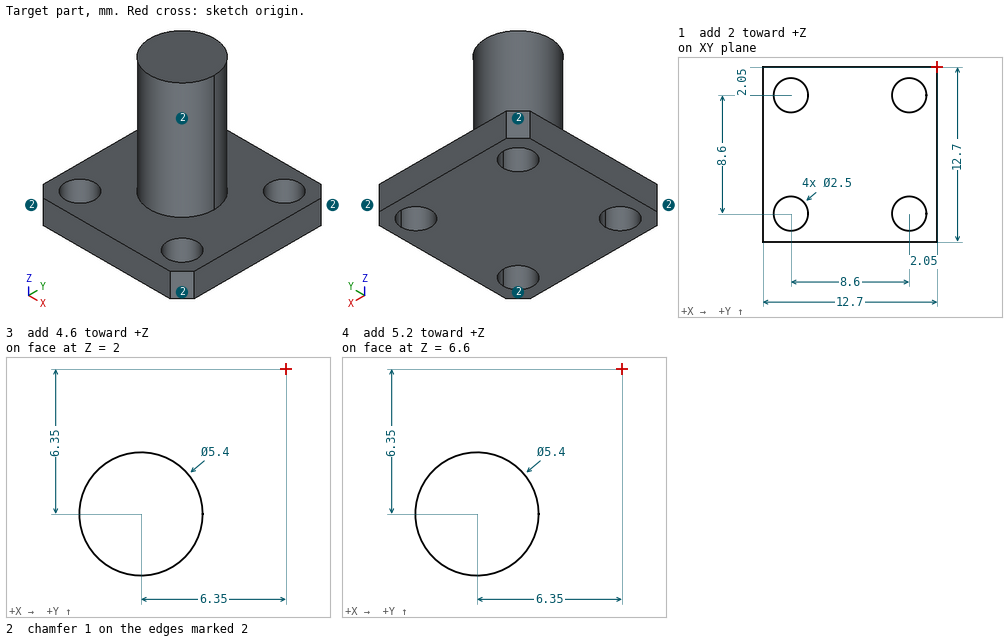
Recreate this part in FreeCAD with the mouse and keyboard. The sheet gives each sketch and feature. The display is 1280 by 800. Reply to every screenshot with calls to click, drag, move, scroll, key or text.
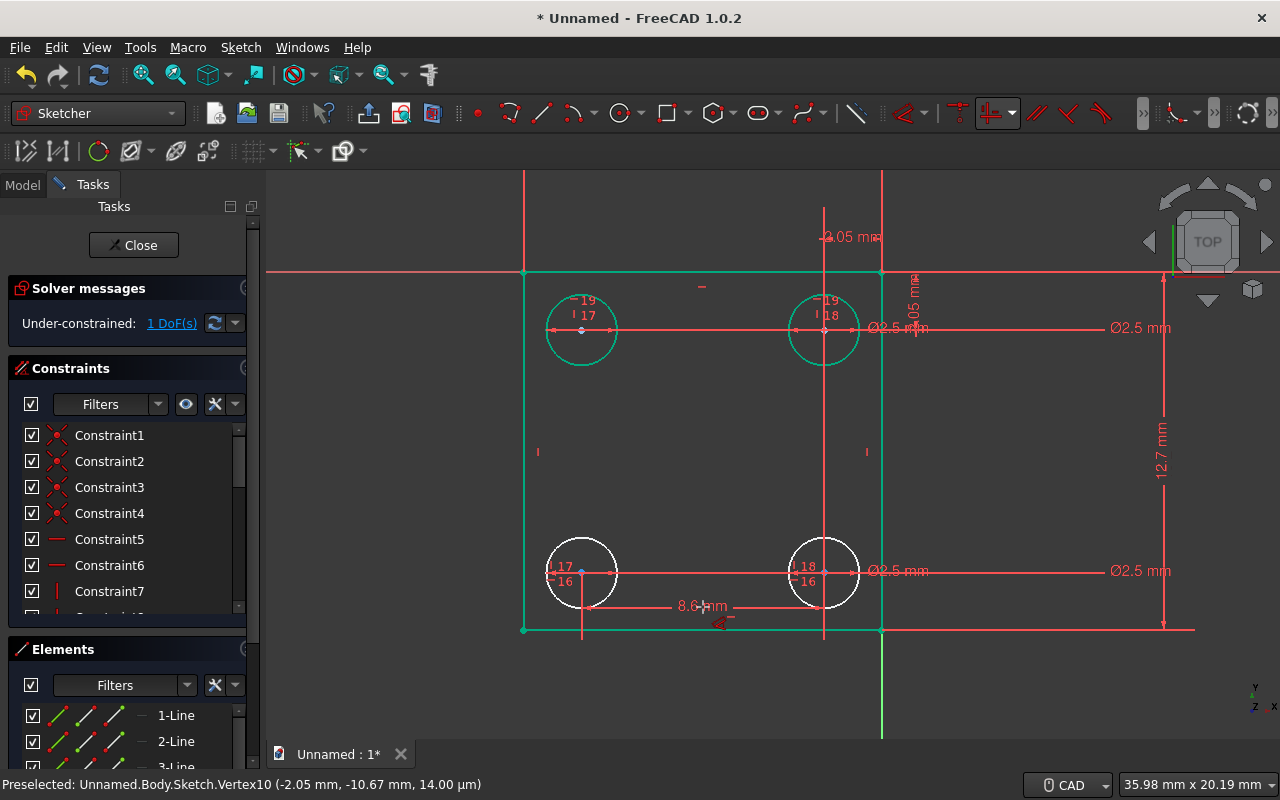
click(582, 573)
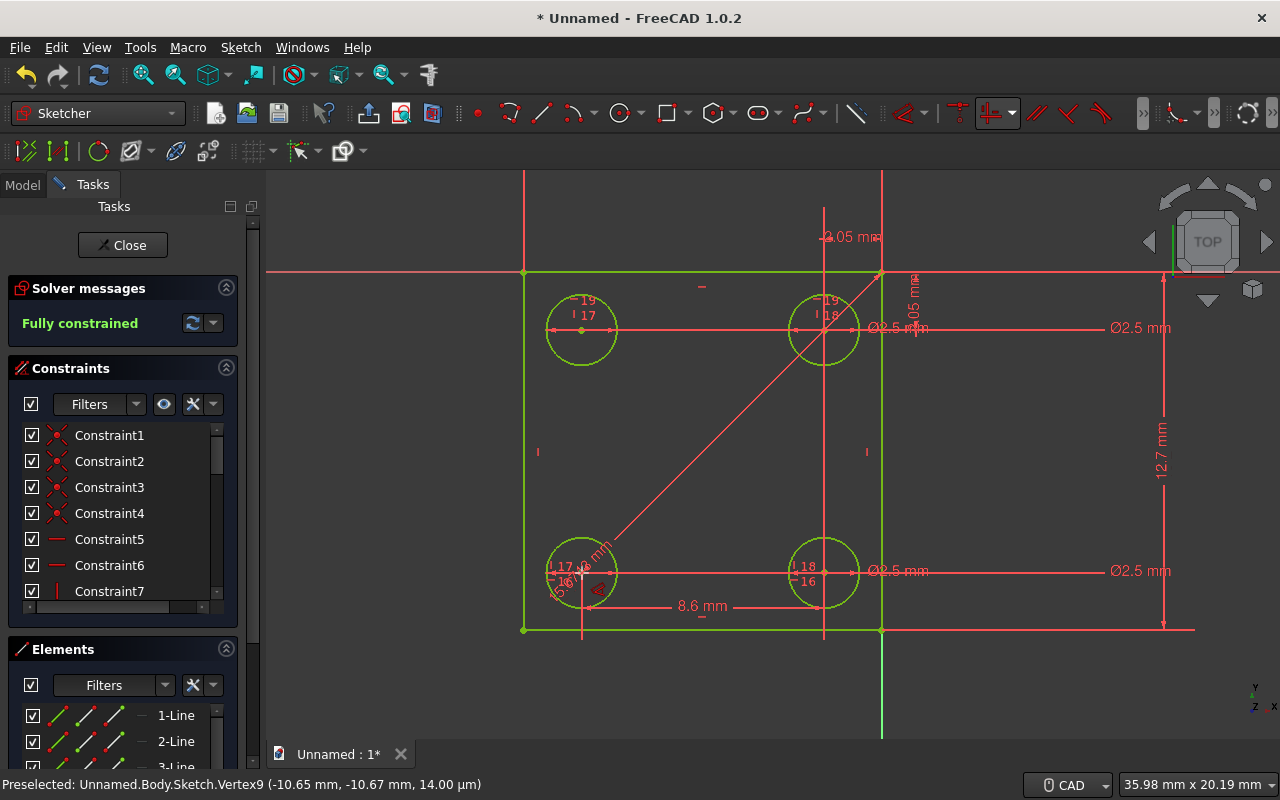
click(582, 330)
click(548, 452)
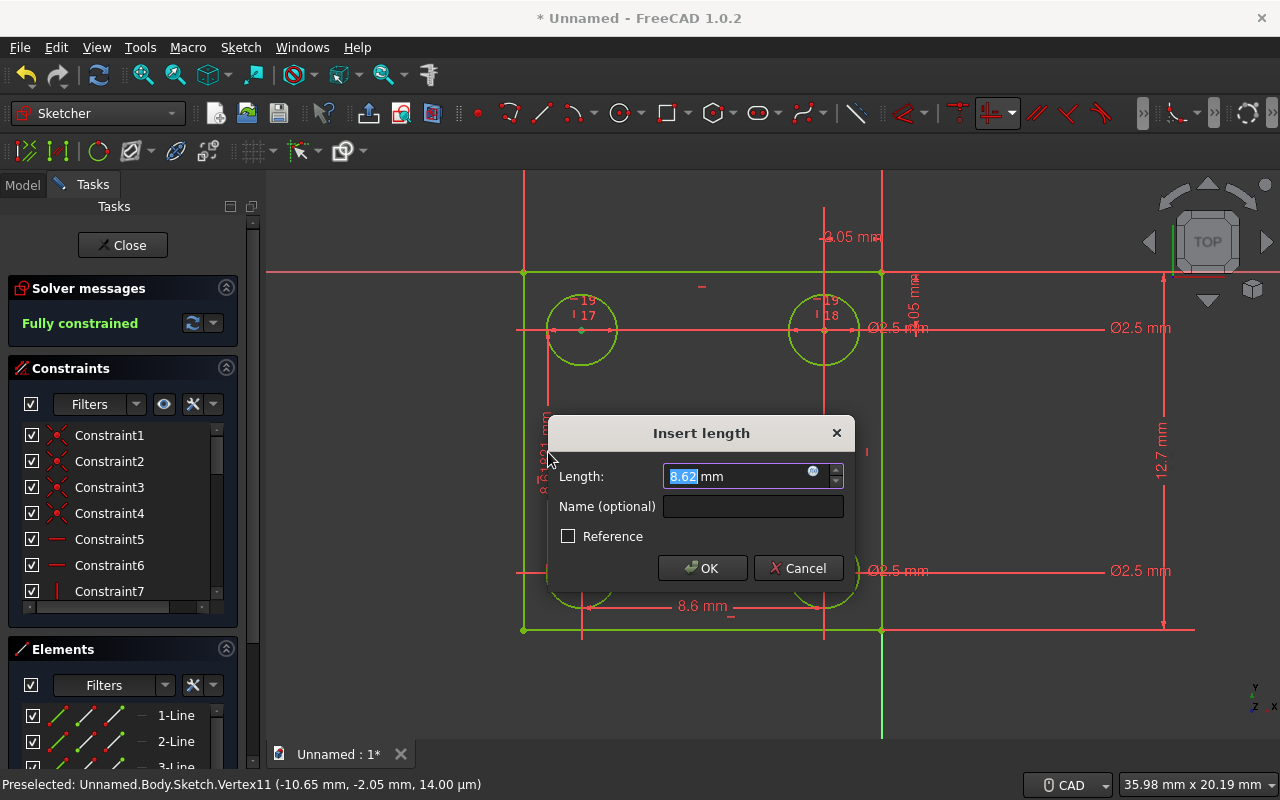
text(8.6)
key(Return)
key(Escape)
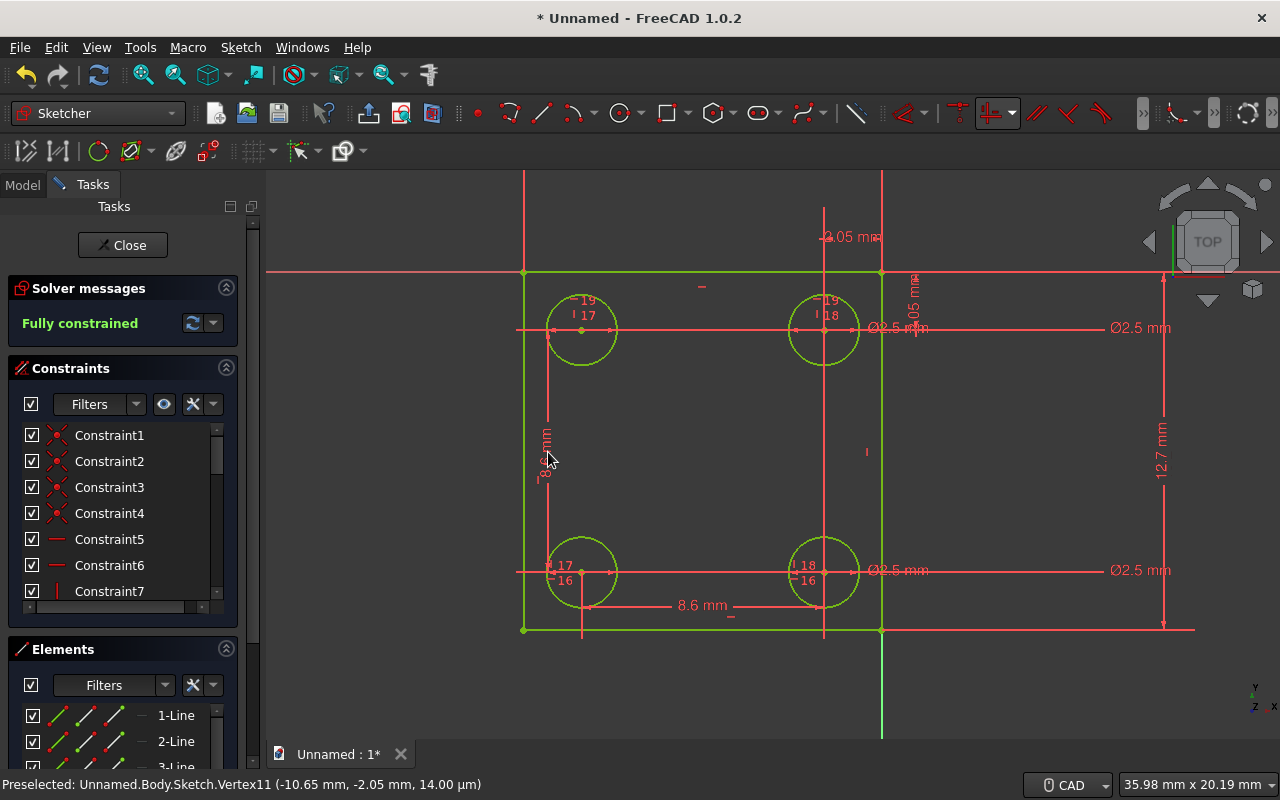
click(123, 245)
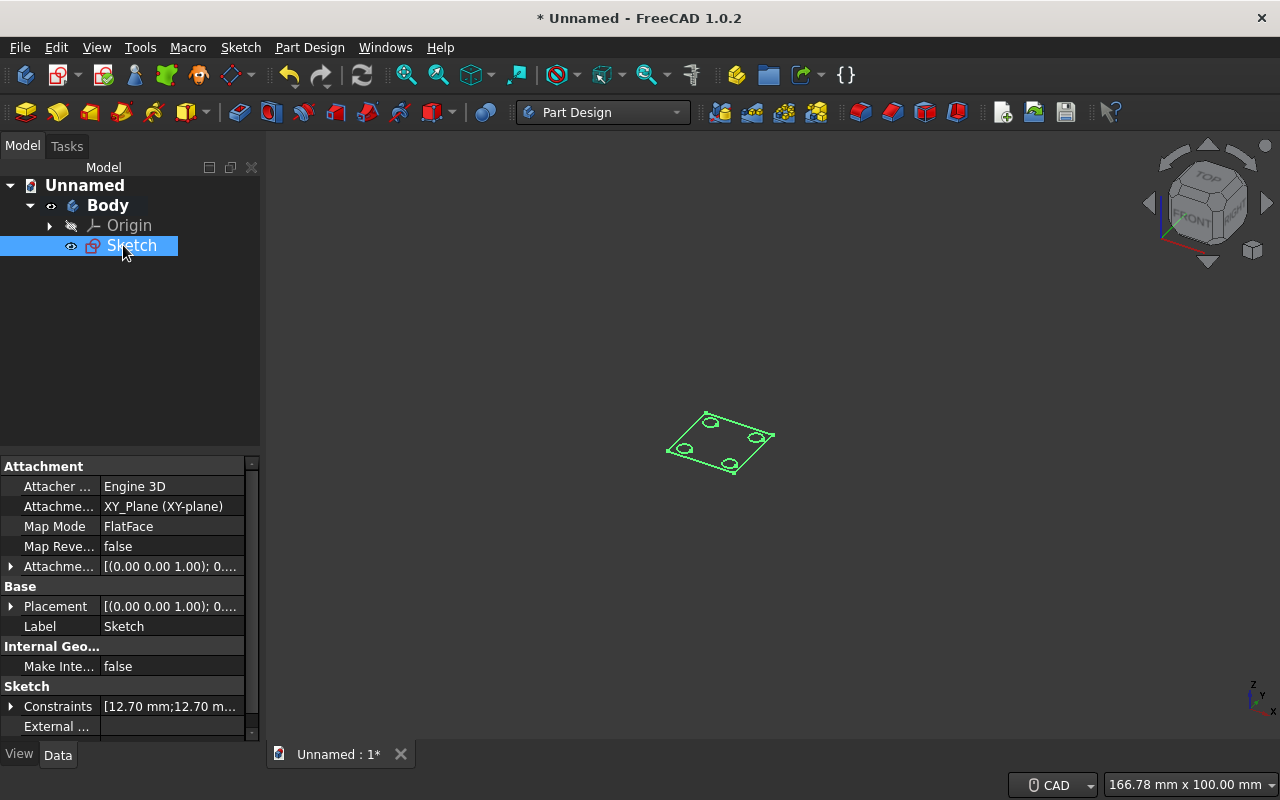
click(26, 112)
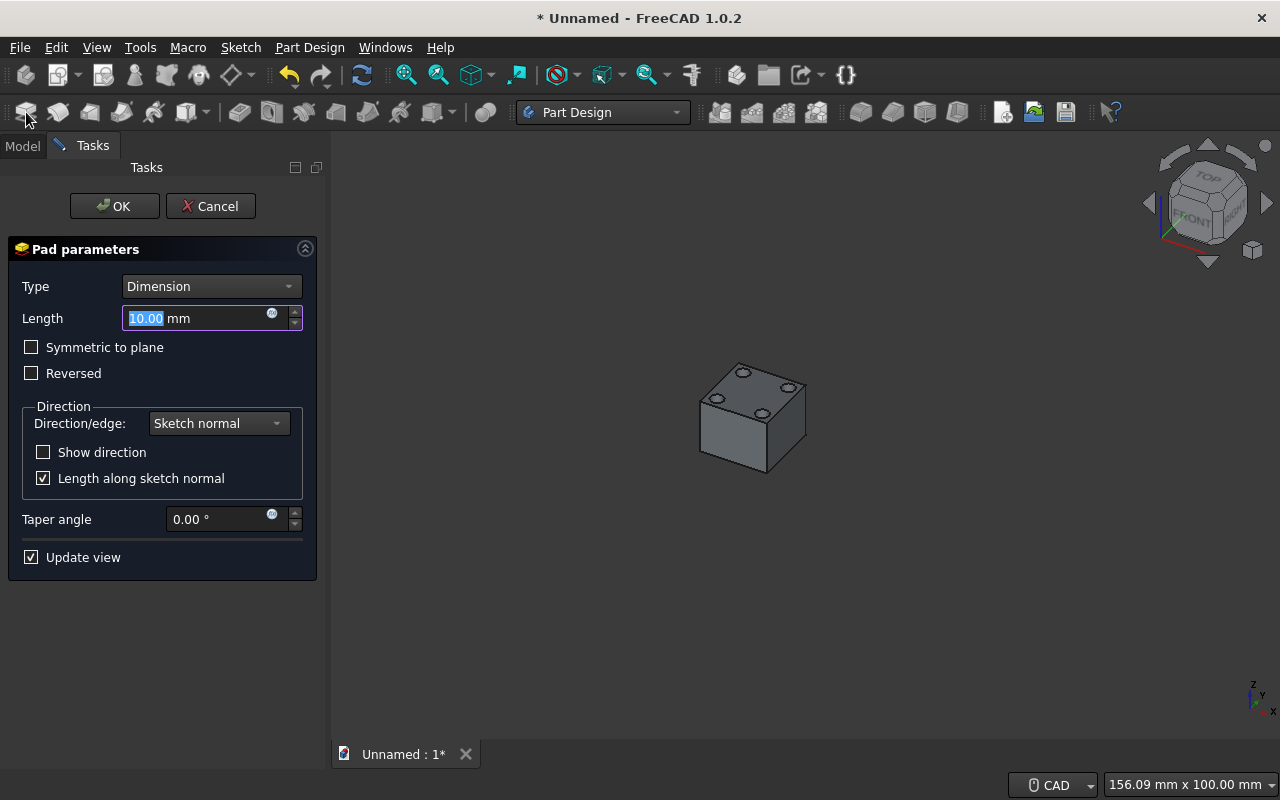
text(2)
key(Tab)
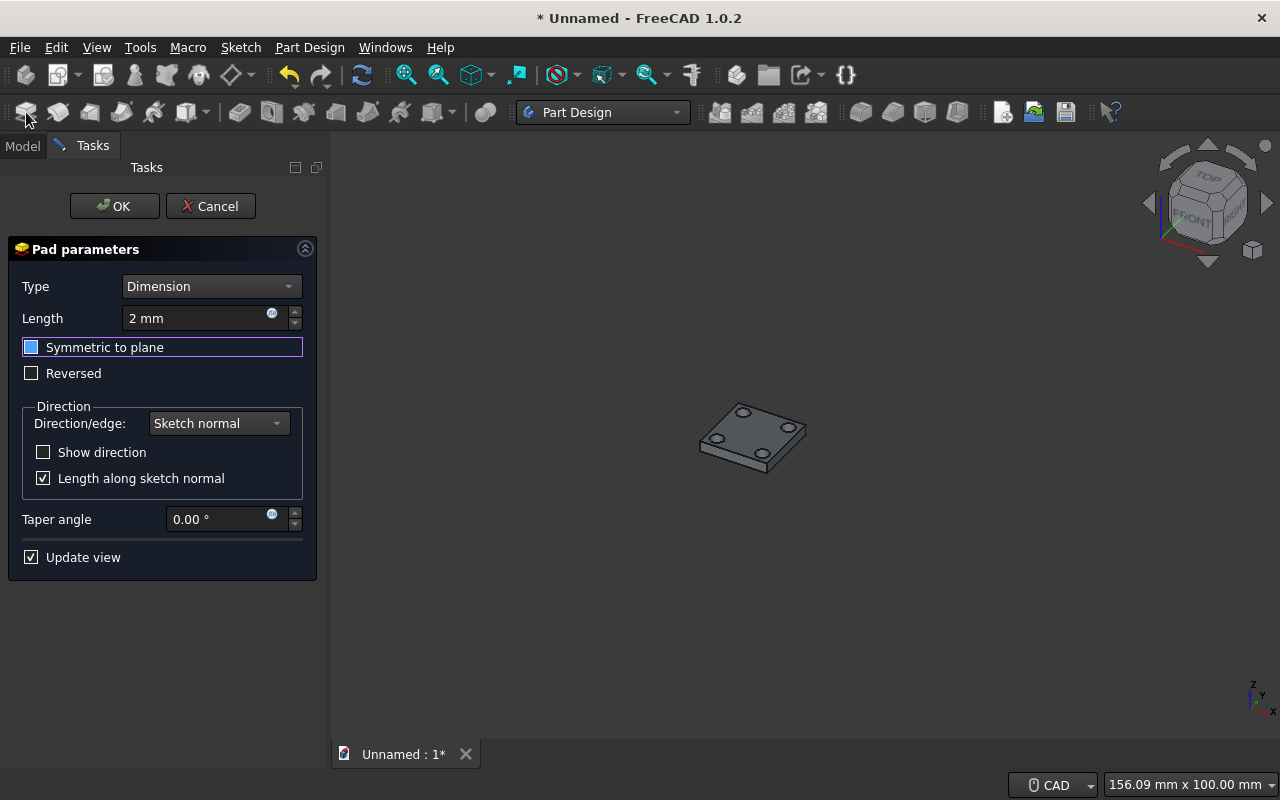
click(115, 206)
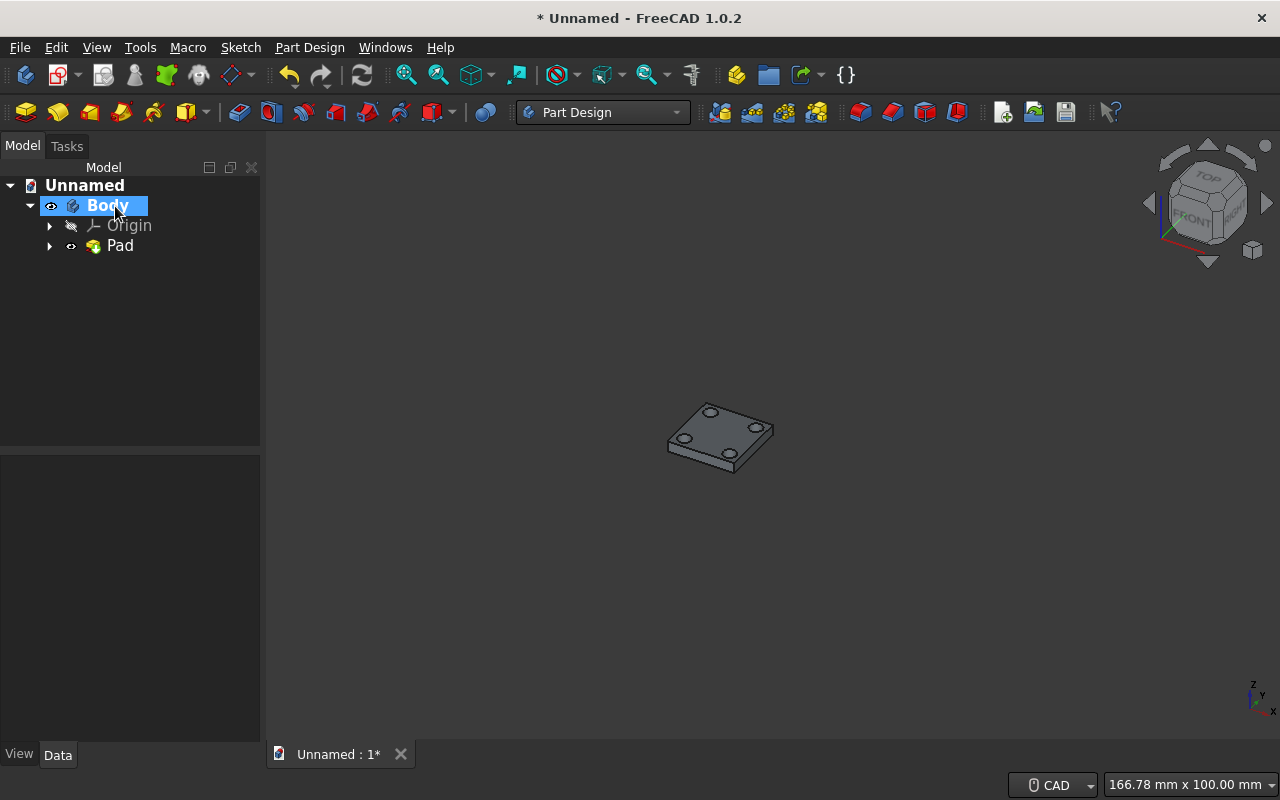
click(408, 76)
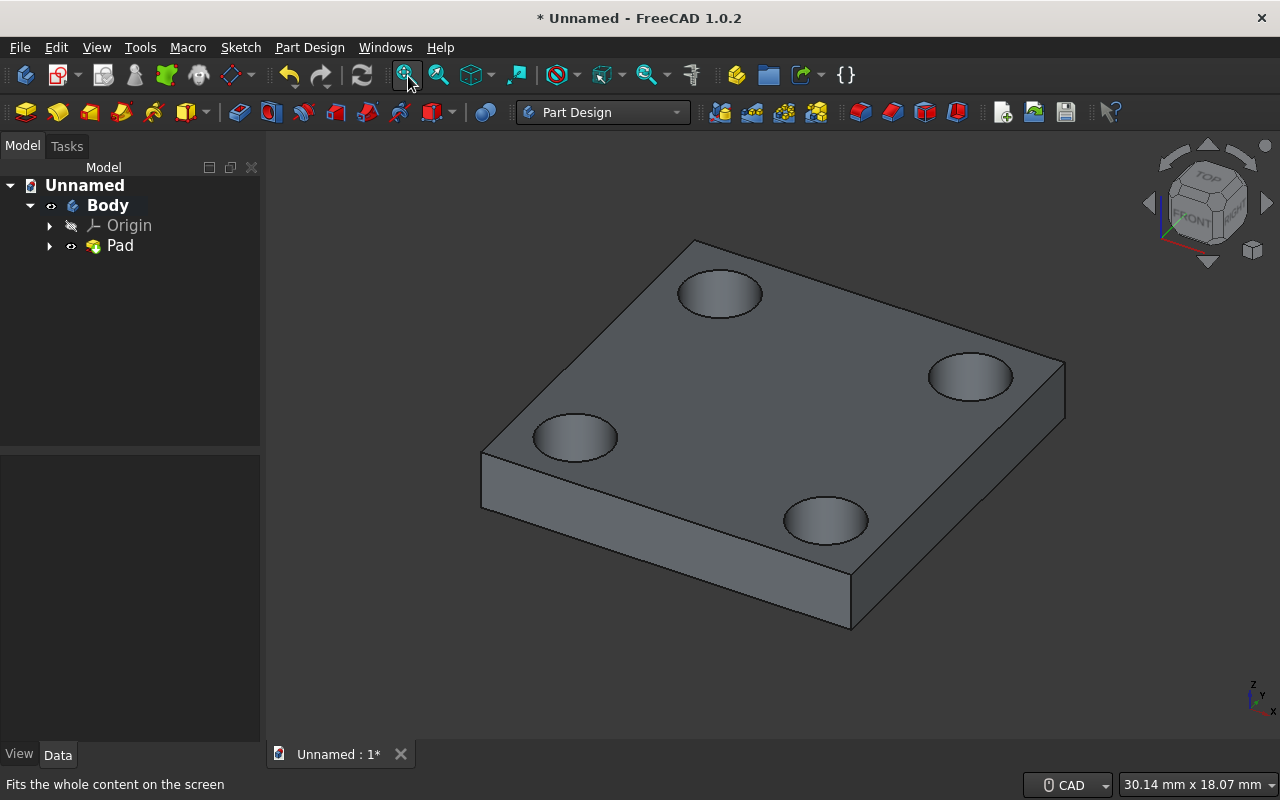
click(851, 601)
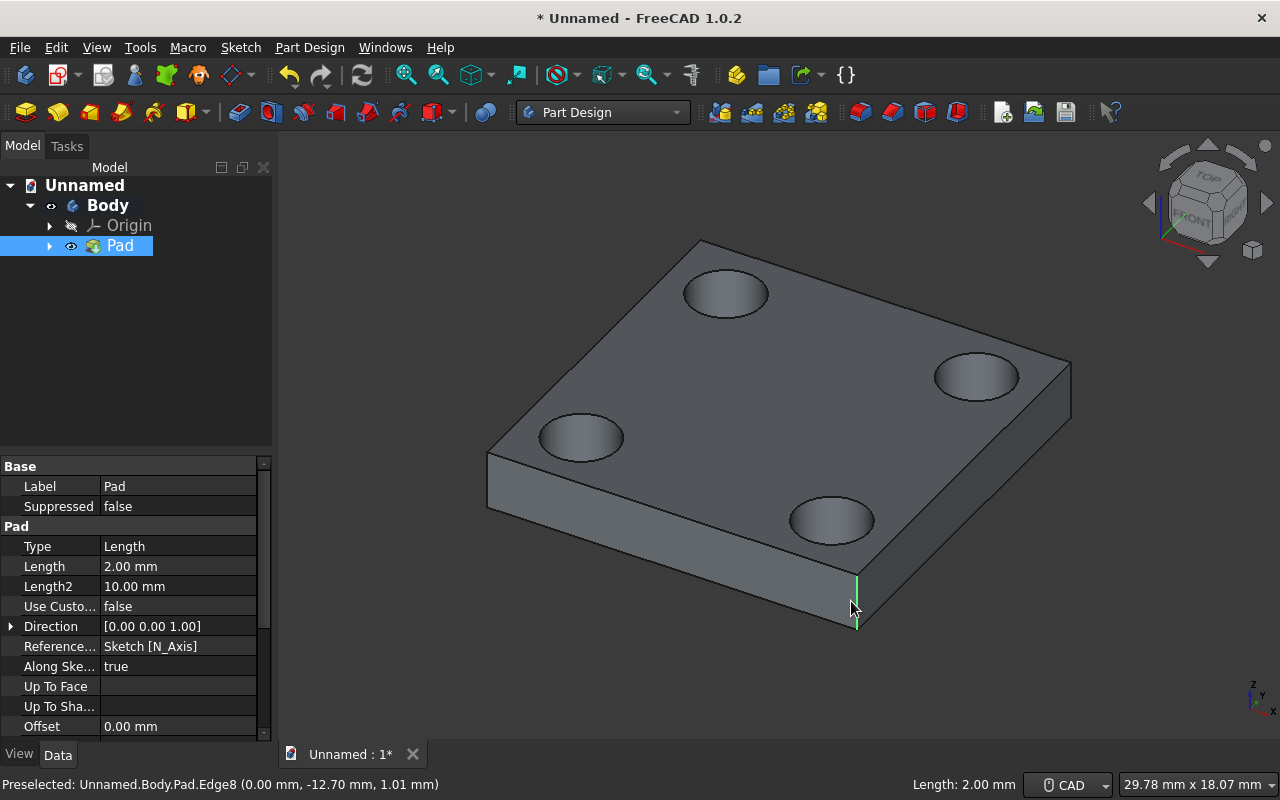
key(0)